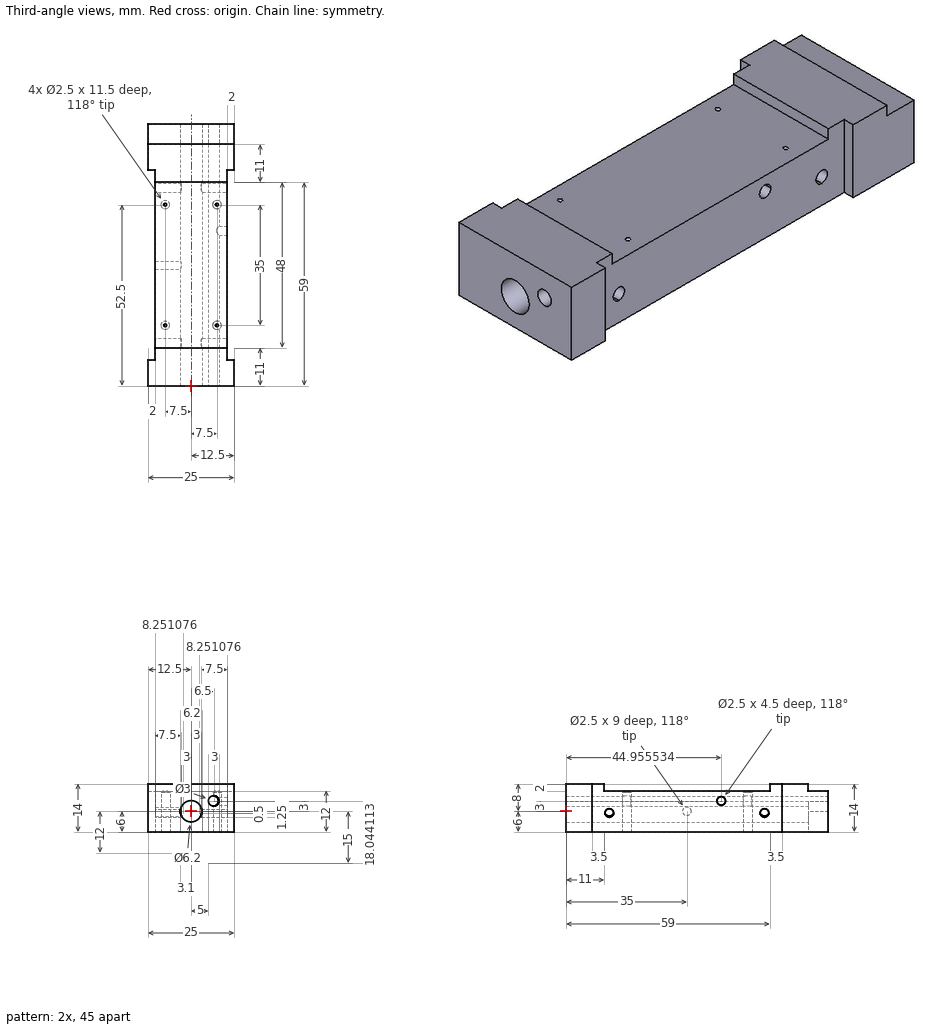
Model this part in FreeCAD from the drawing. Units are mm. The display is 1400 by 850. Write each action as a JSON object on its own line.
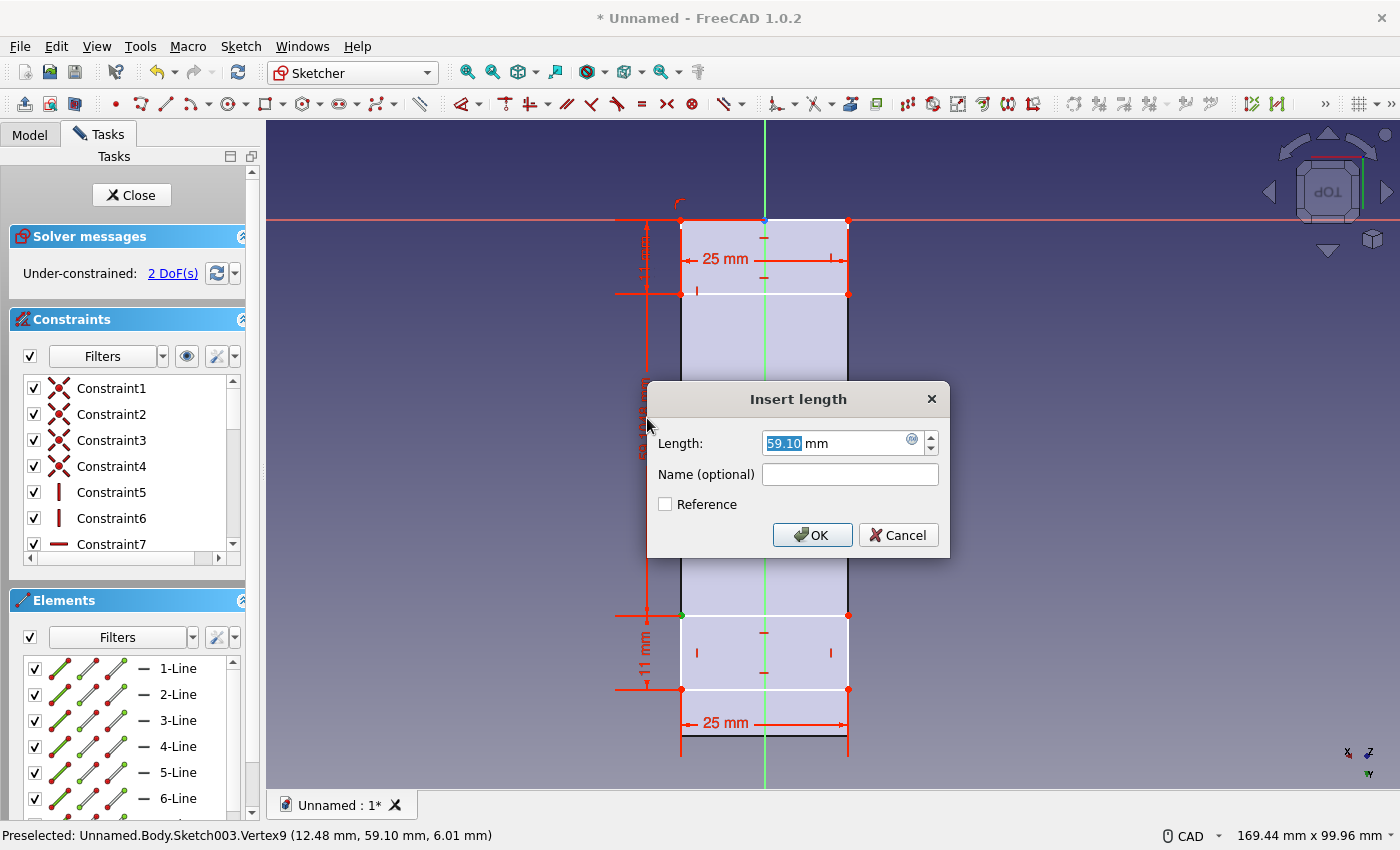
{"action": "type", "text": "59"}
{"action": "key", "text": "Return"}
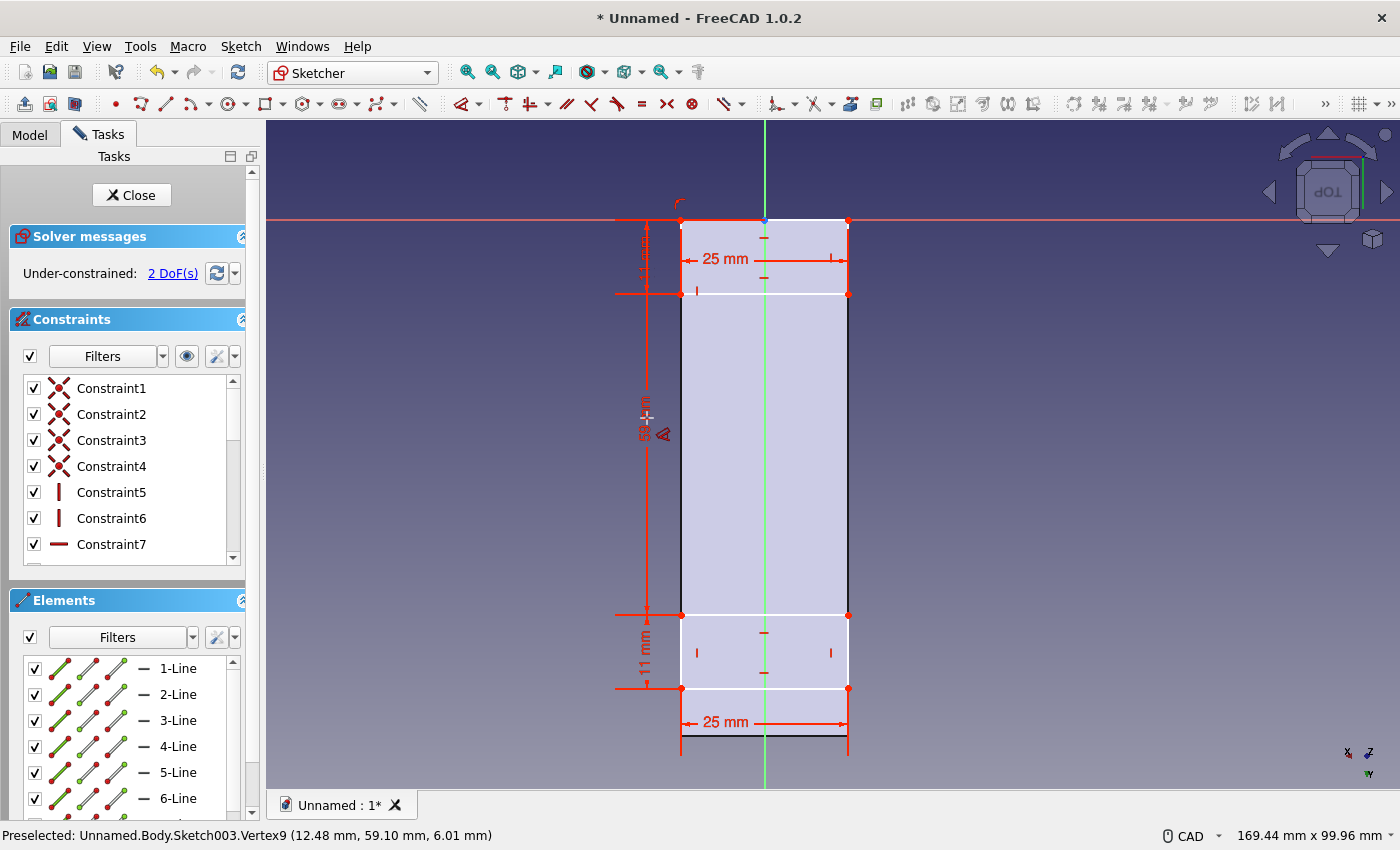
{"action": "left_click", "coordinate": [681, 220]}
{"action": "left_click", "coordinate": [723, 186]}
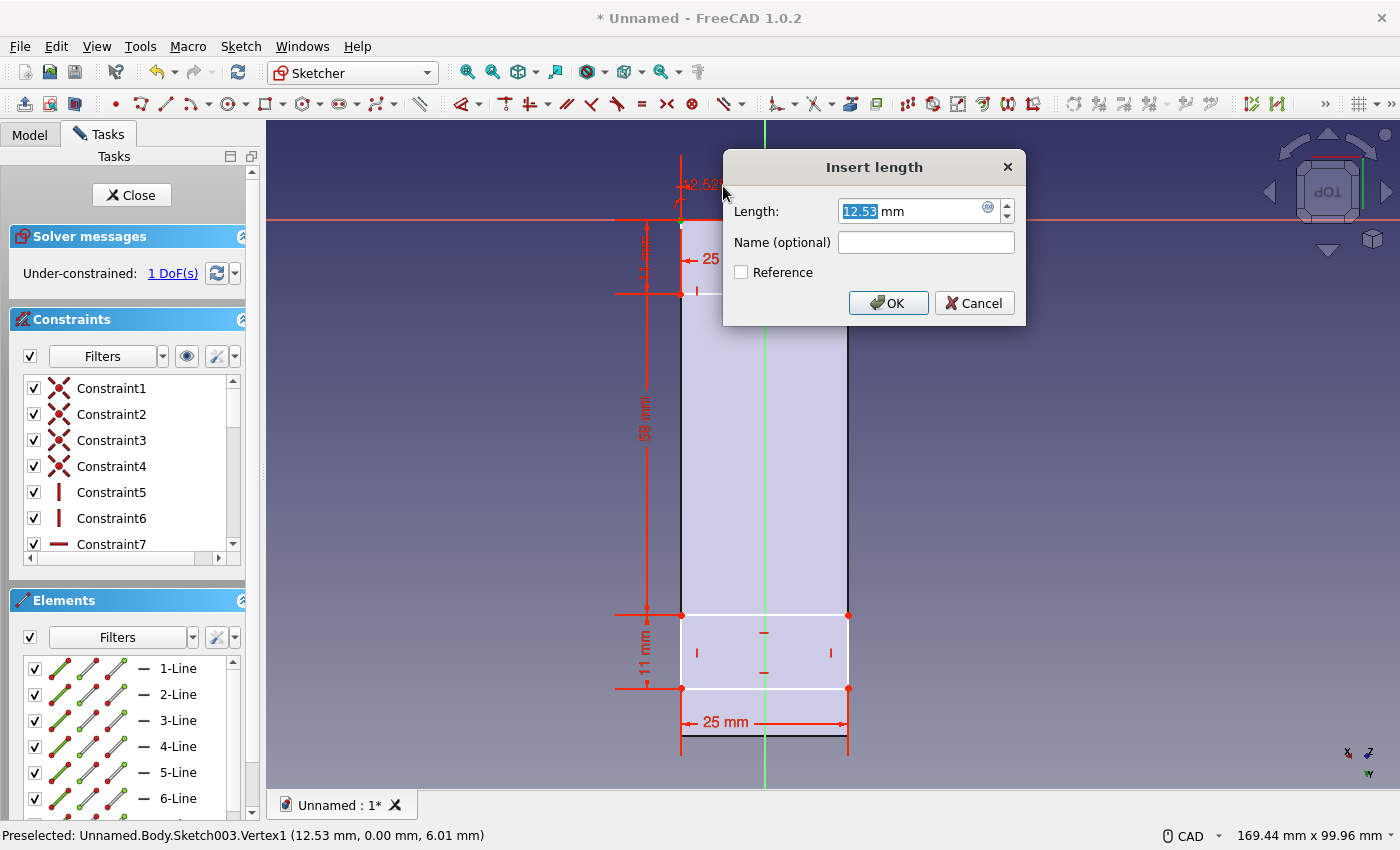
{"action": "type", "text": "12.5"}
{"action": "key", "text": "Return"}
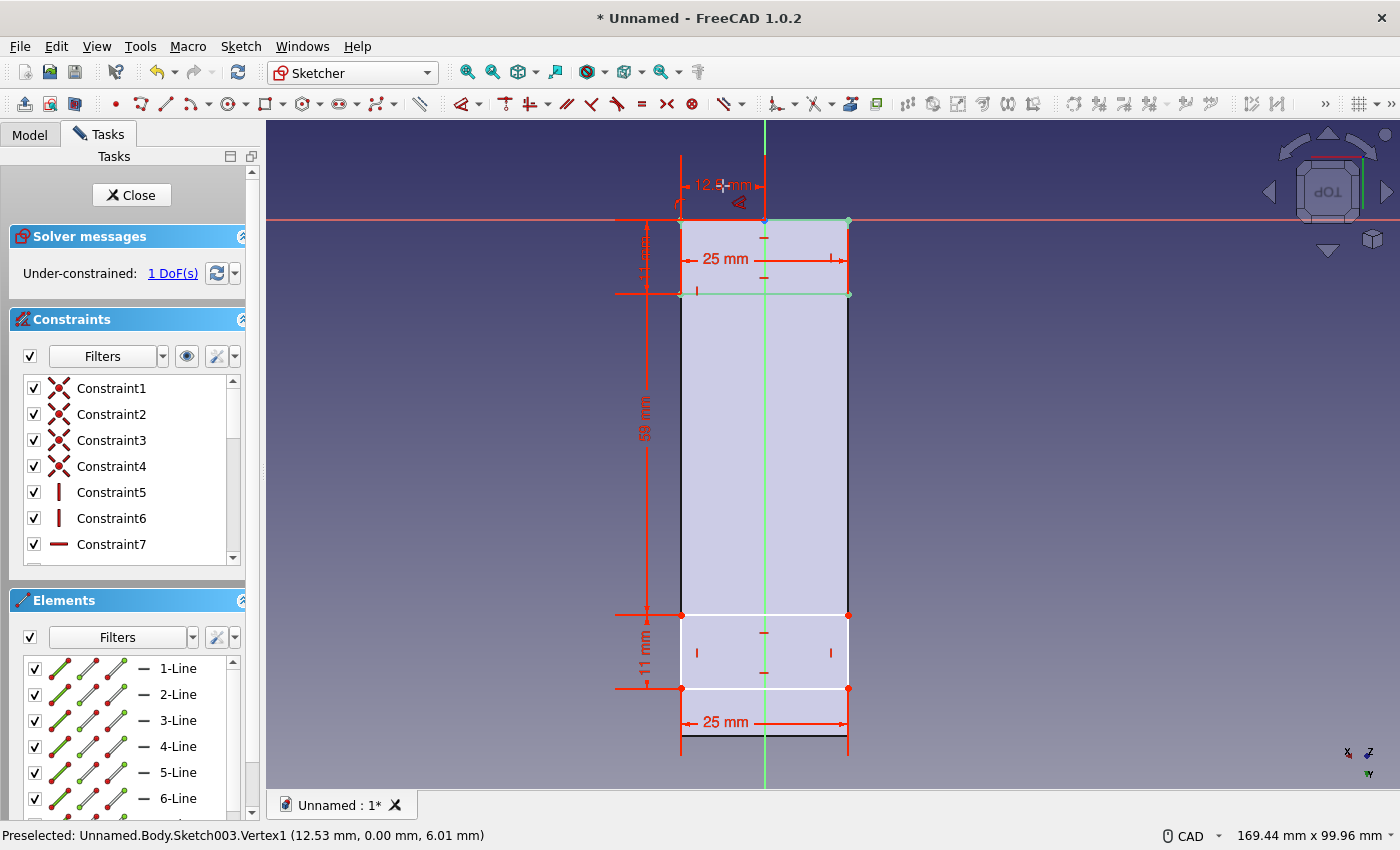
{"action": "left_click", "coordinate": [681, 615]}
{"action": "left_click", "coordinate": [723, 649]}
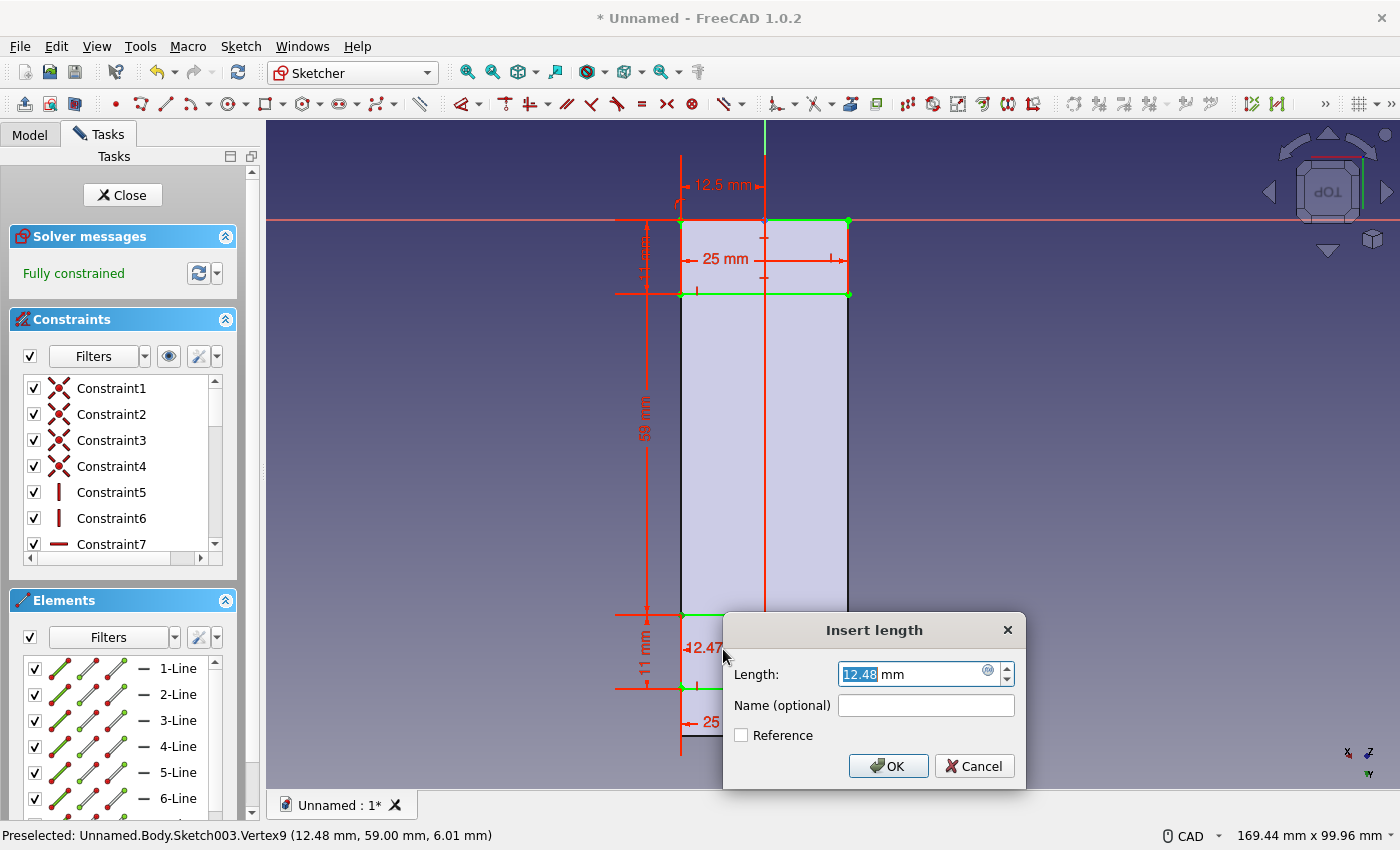
{"action": "type", "text": "12.5"}
{"action": "key", "text": "Return"}
{"action": "key", "text": "Escape"}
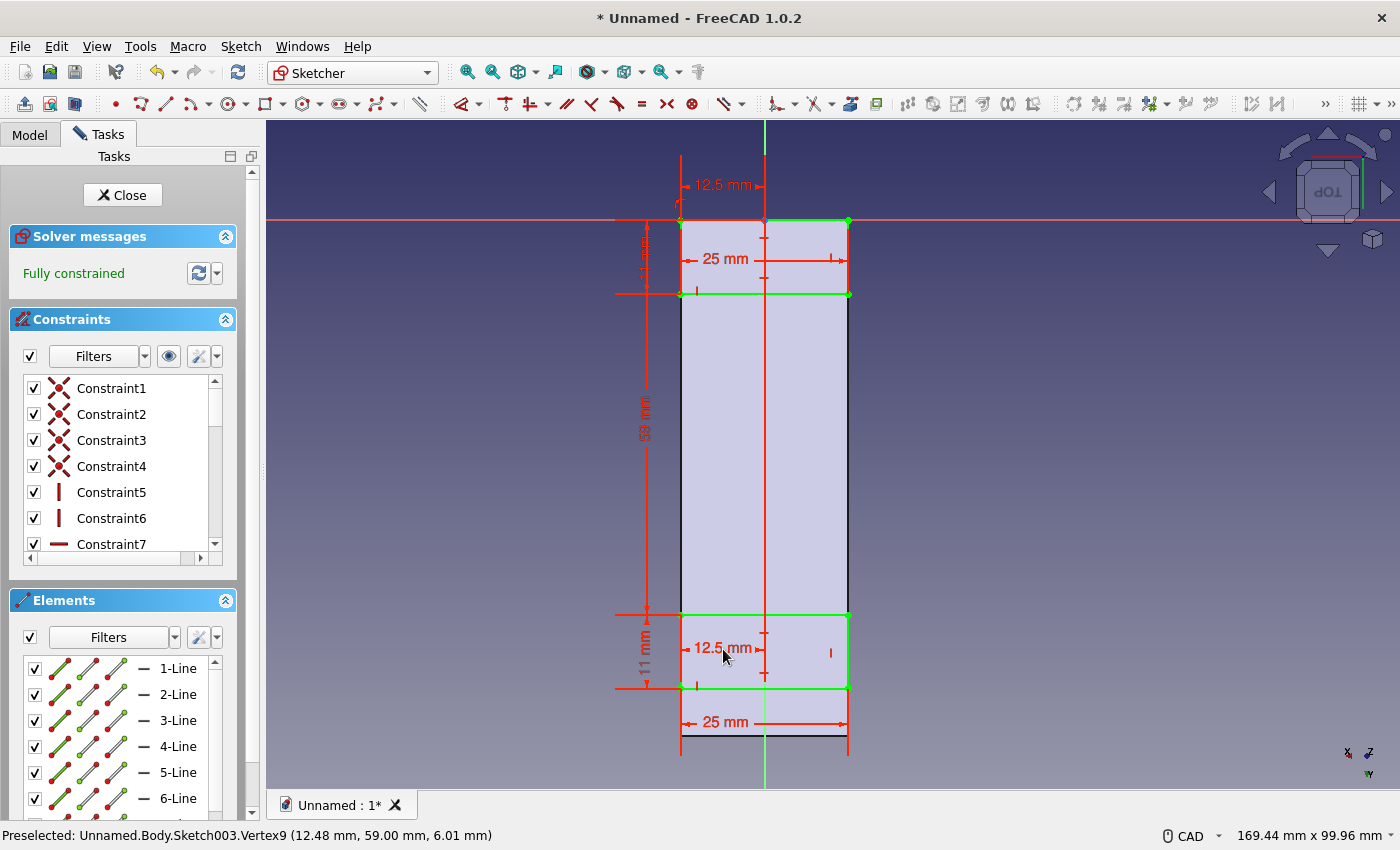
{"action": "left_click", "coordinate": [123, 195]}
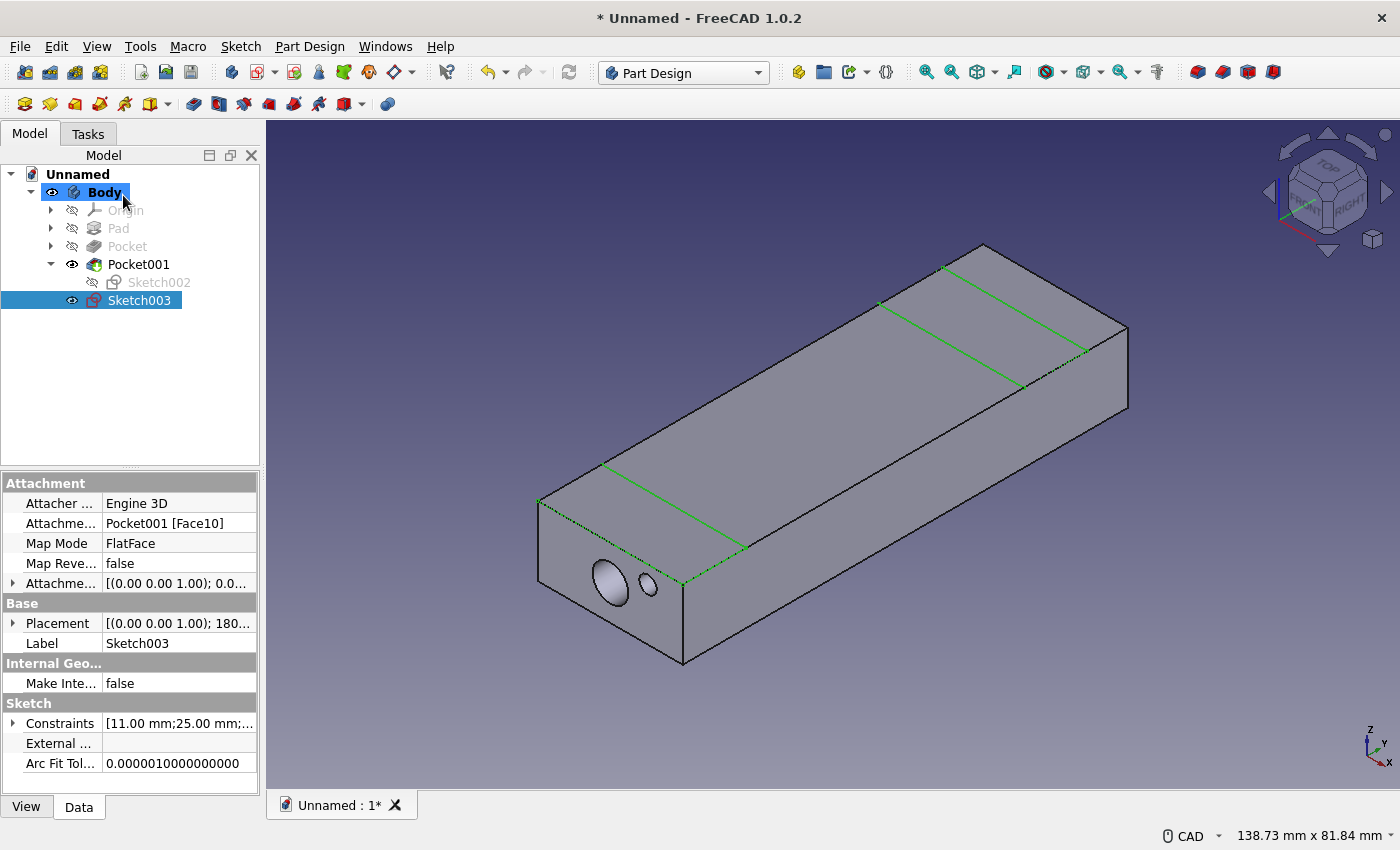
{"action": "left_click", "coordinate": [25, 104]}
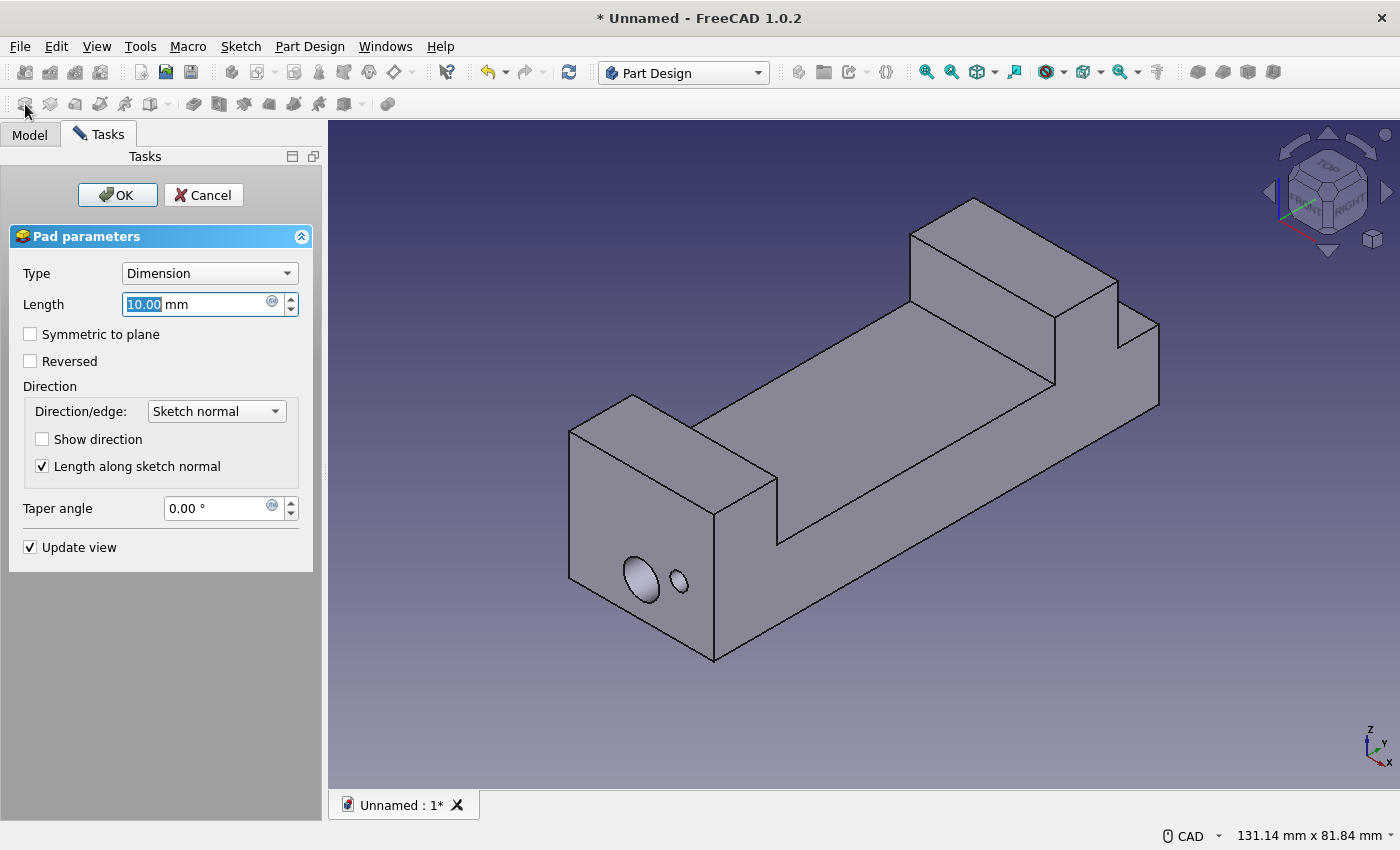
{"action": "type", "text": "2"}
{"action": "key", "text": "Tab"}